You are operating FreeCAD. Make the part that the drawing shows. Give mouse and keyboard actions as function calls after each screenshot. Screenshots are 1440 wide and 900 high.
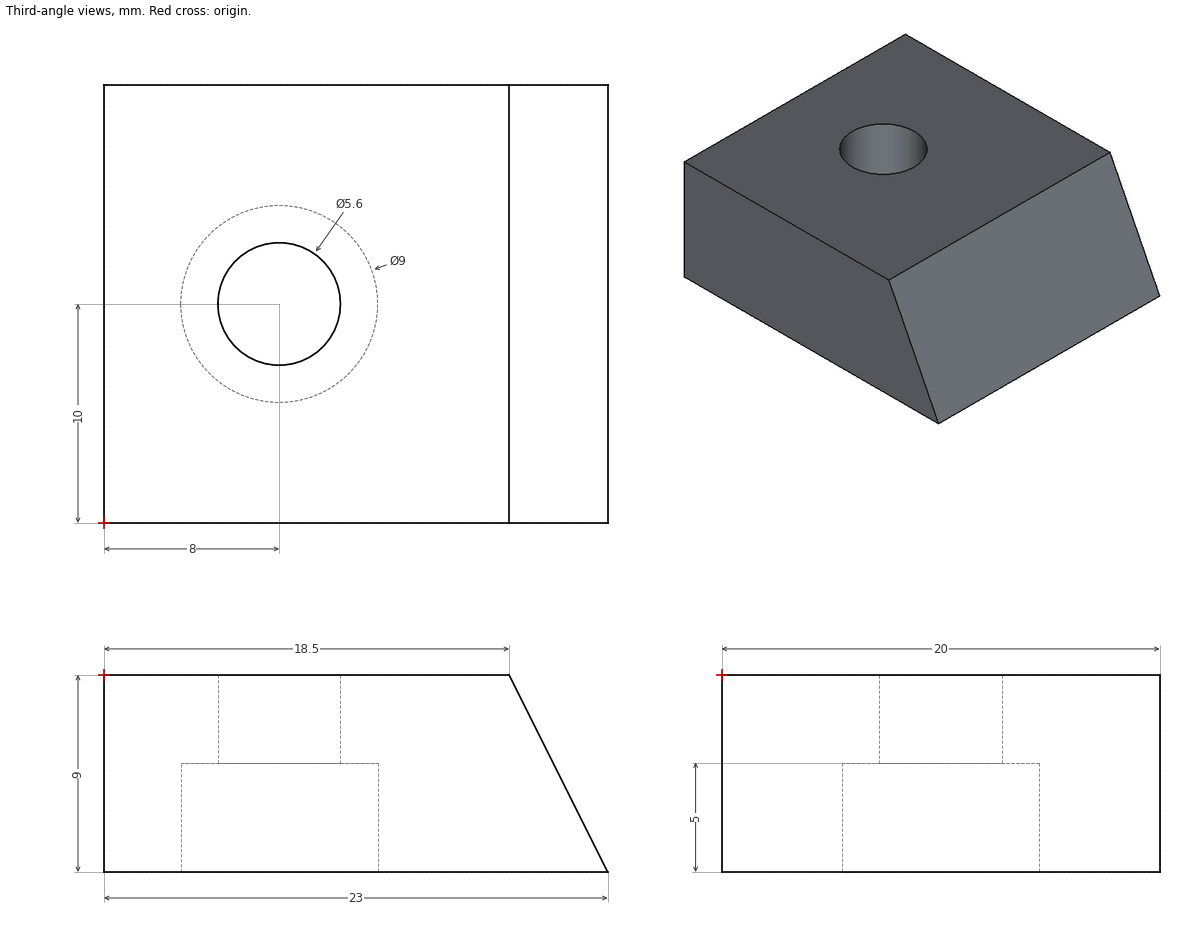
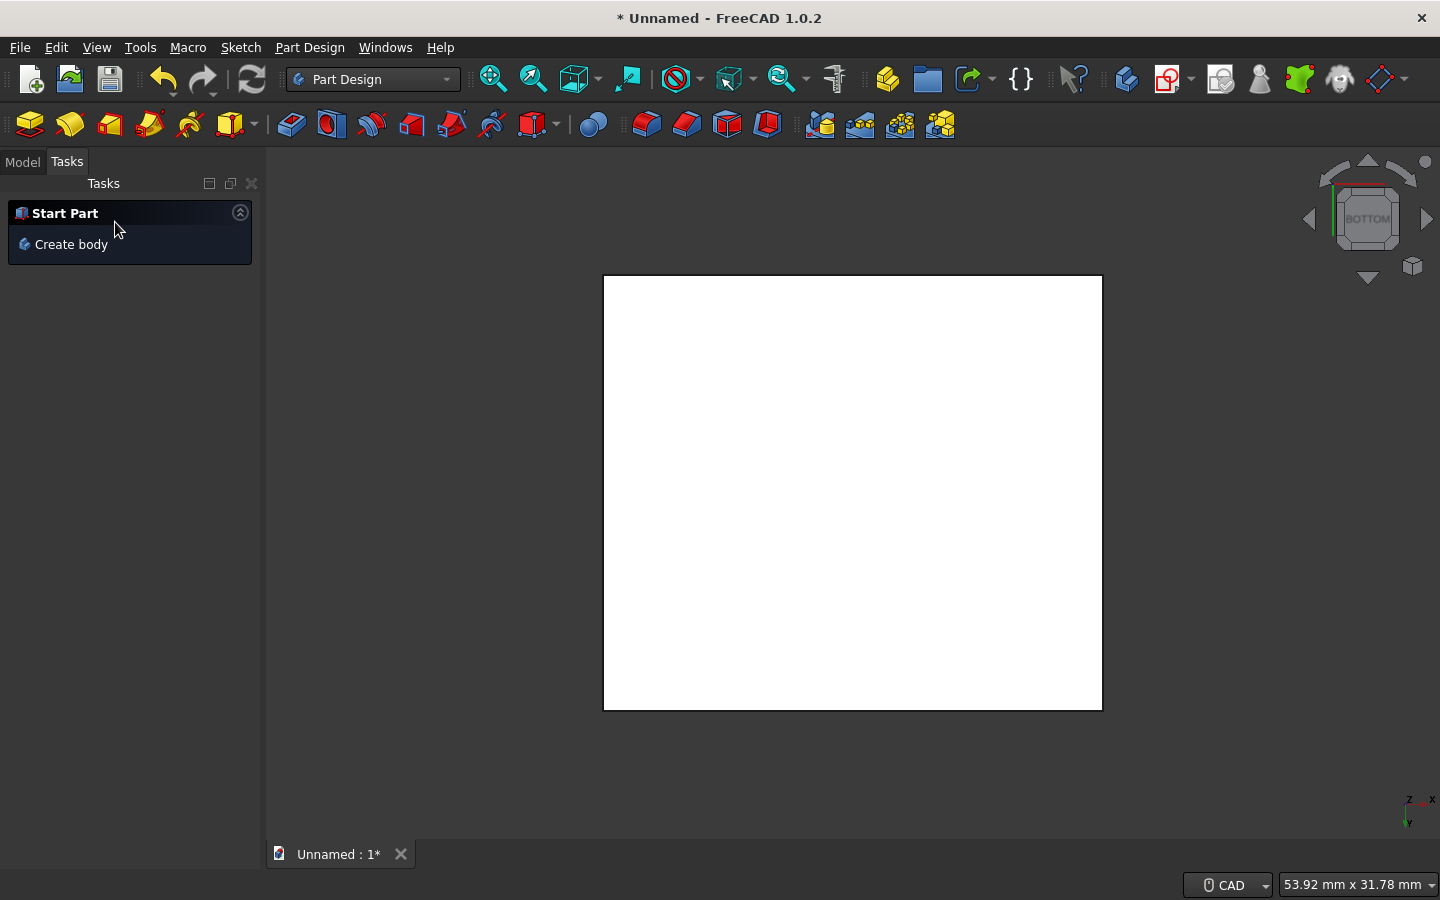
click(853, 492)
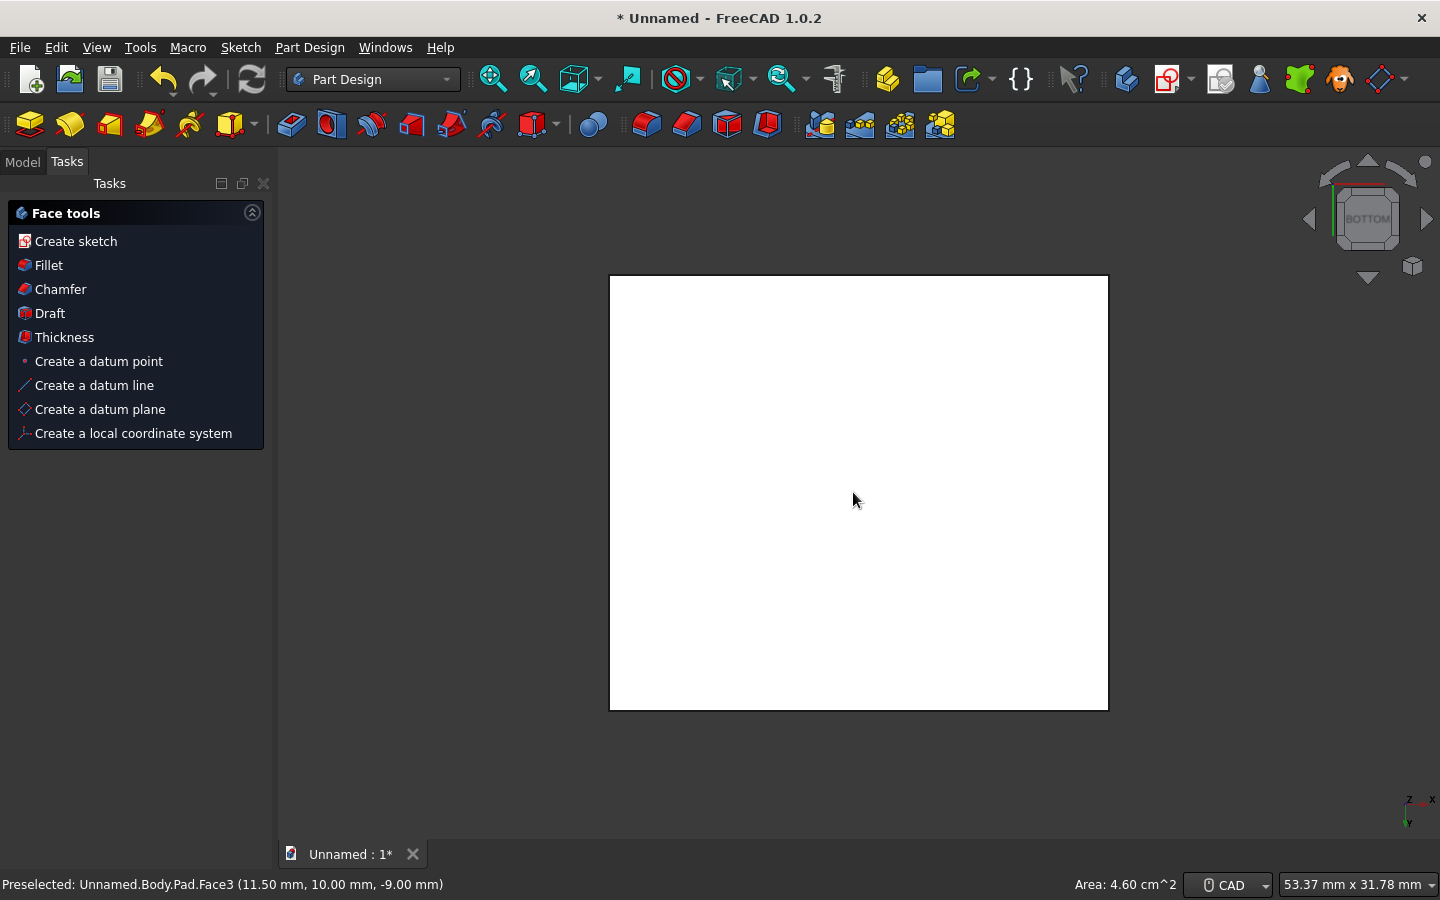
click(1168, 80)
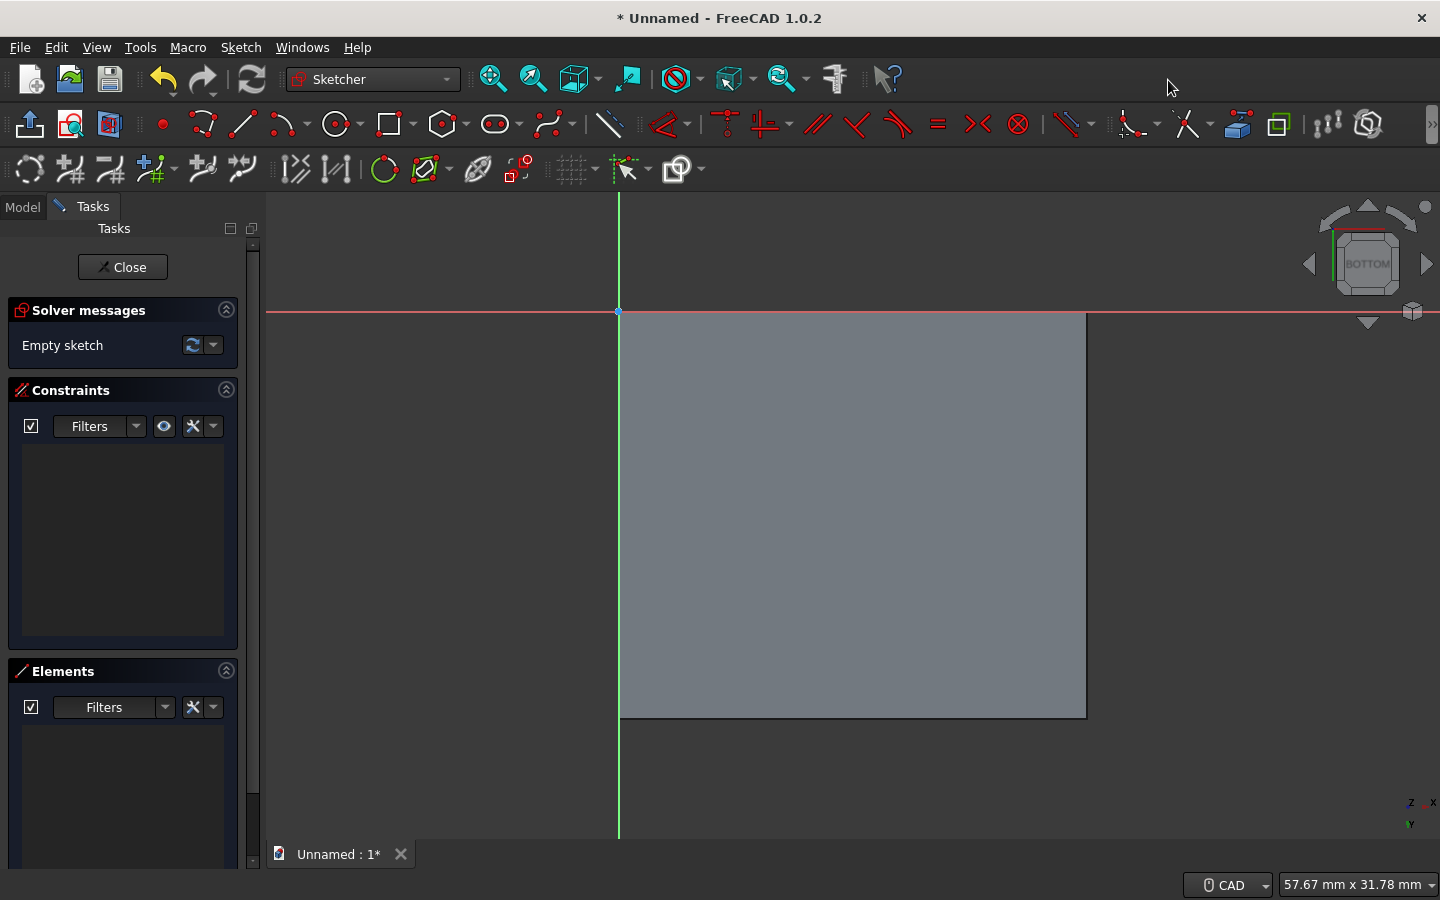
scroll(668, 346, up, 2)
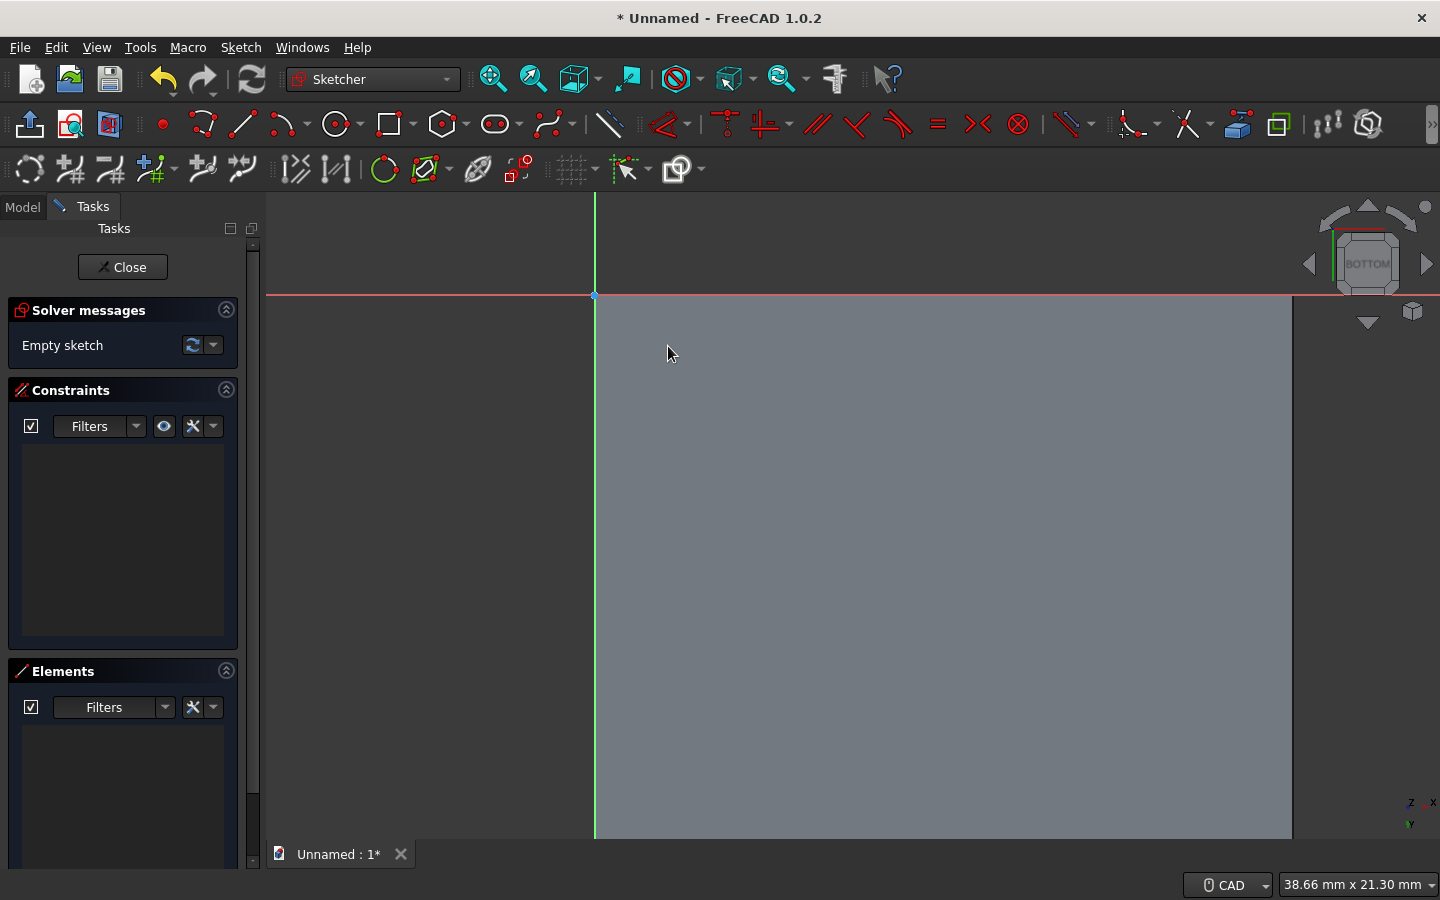
click(336, 124)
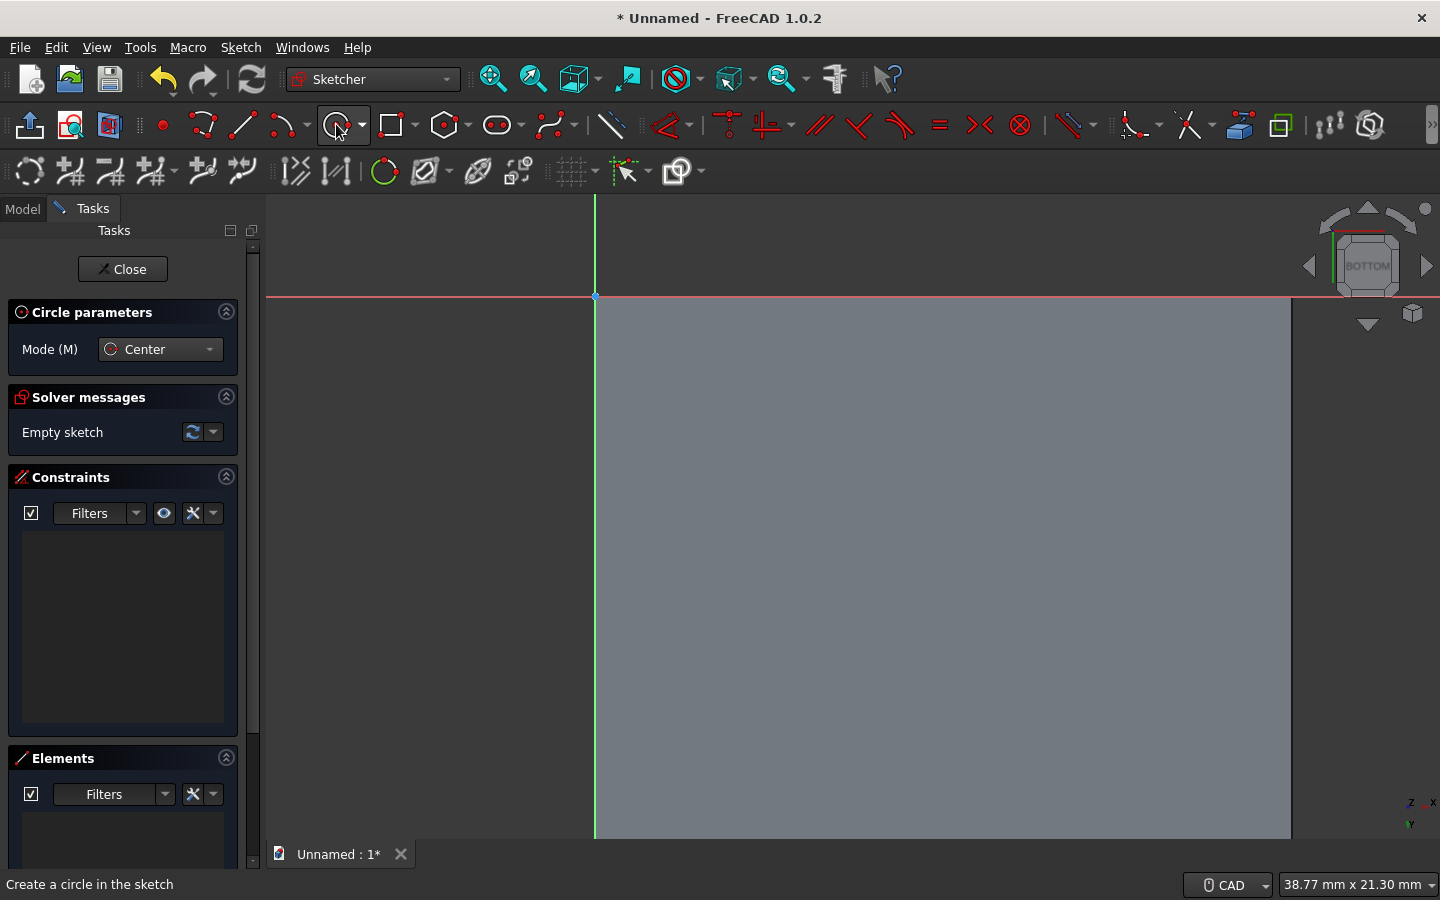
click(838, 599)
move(934, 503)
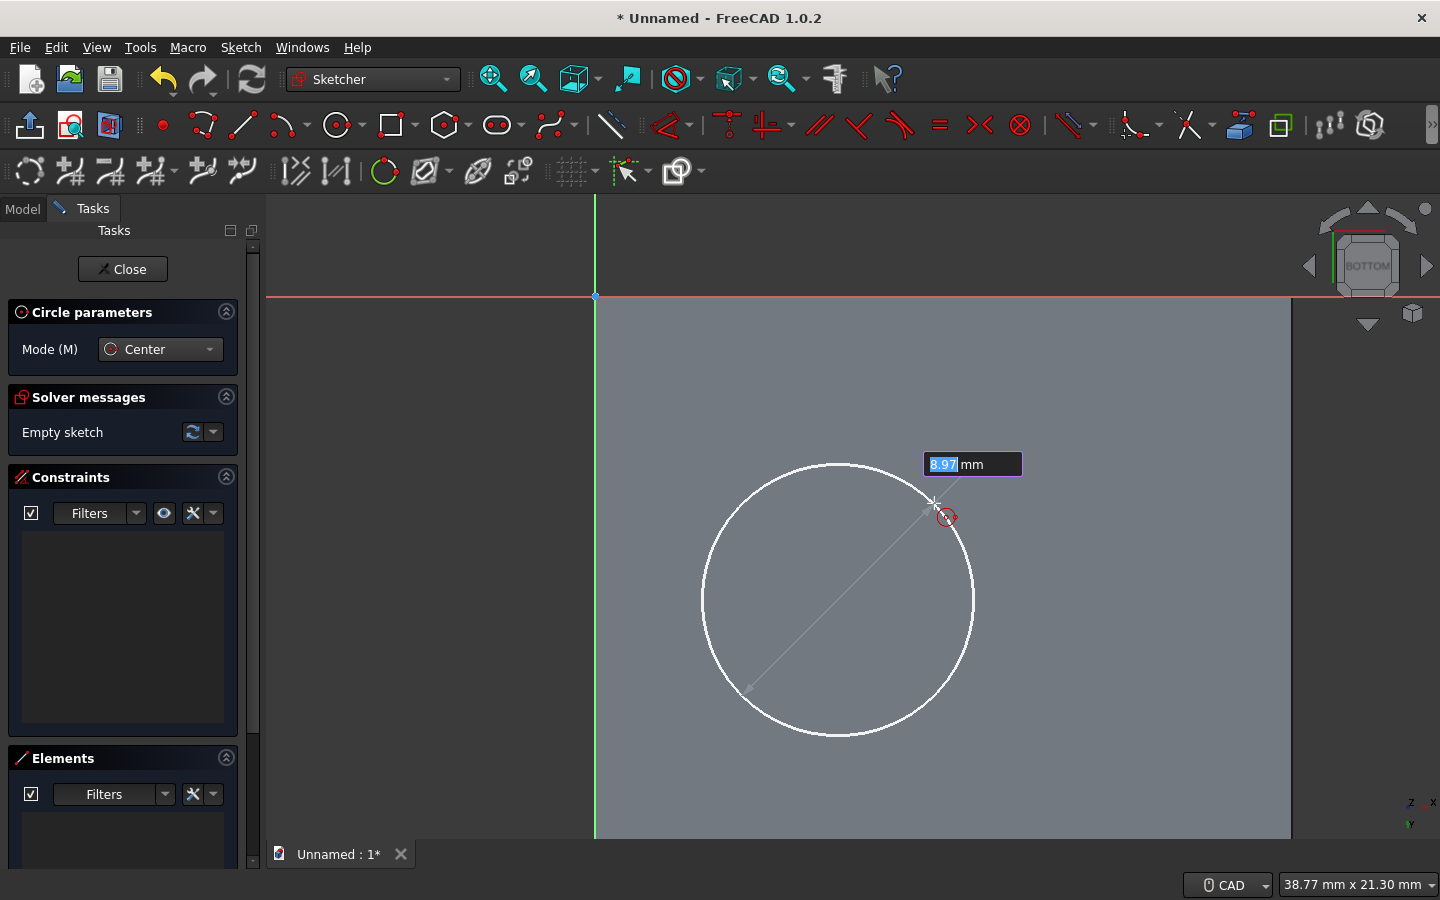
text(9)
key(Return)
key(Escape)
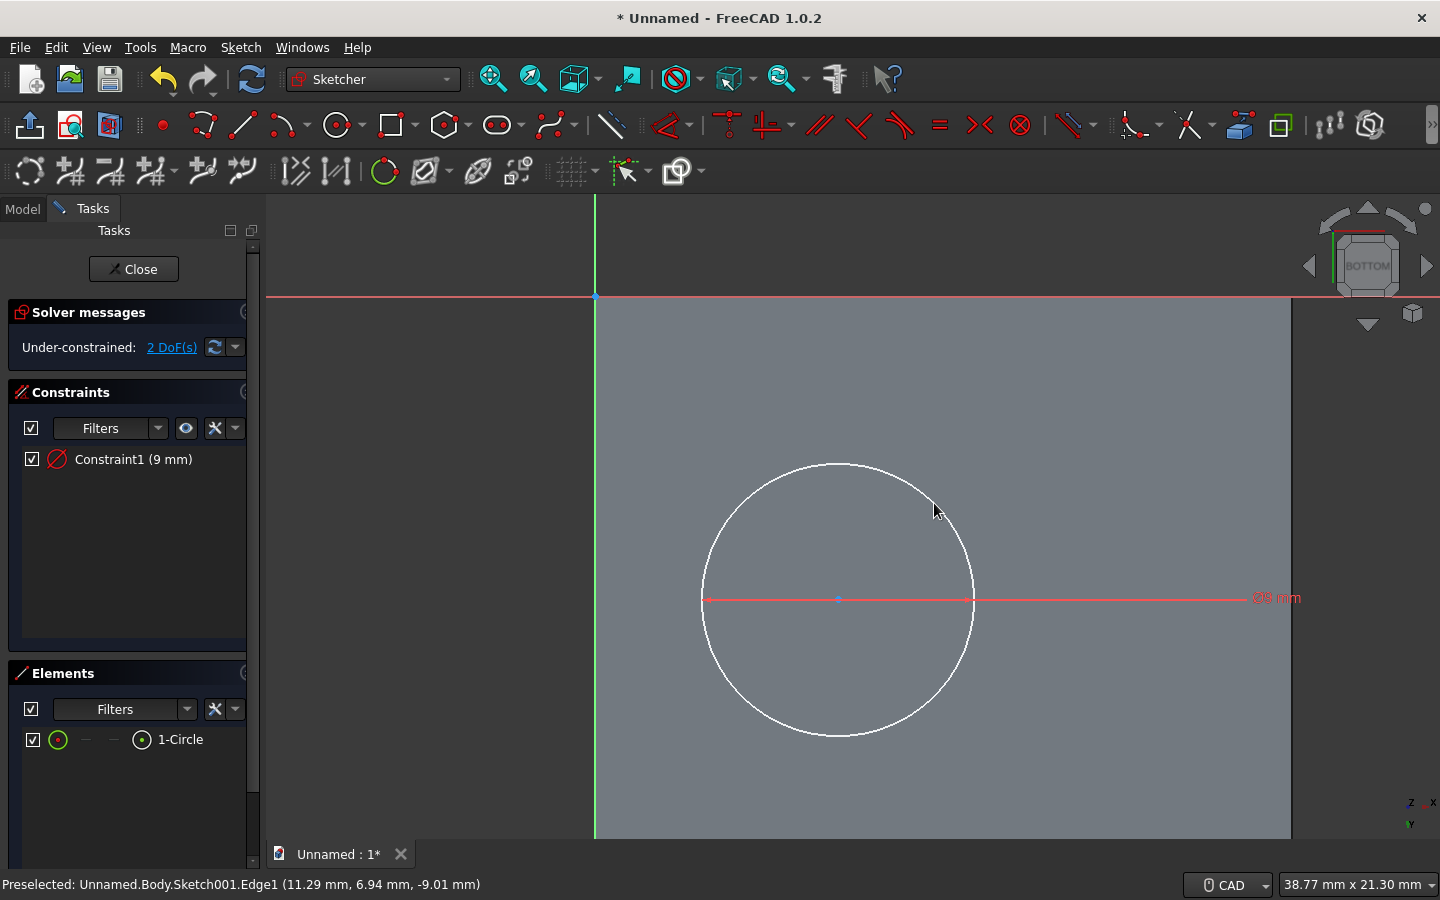
click(666, 126)